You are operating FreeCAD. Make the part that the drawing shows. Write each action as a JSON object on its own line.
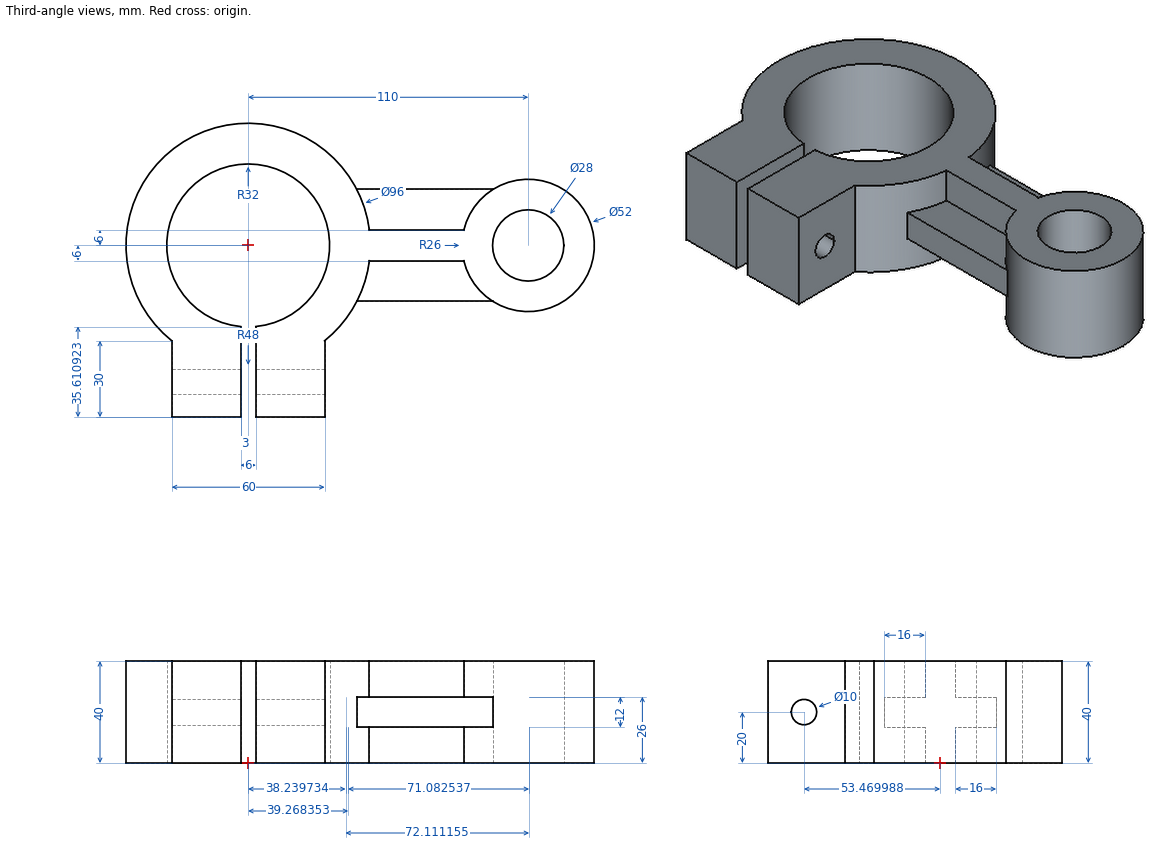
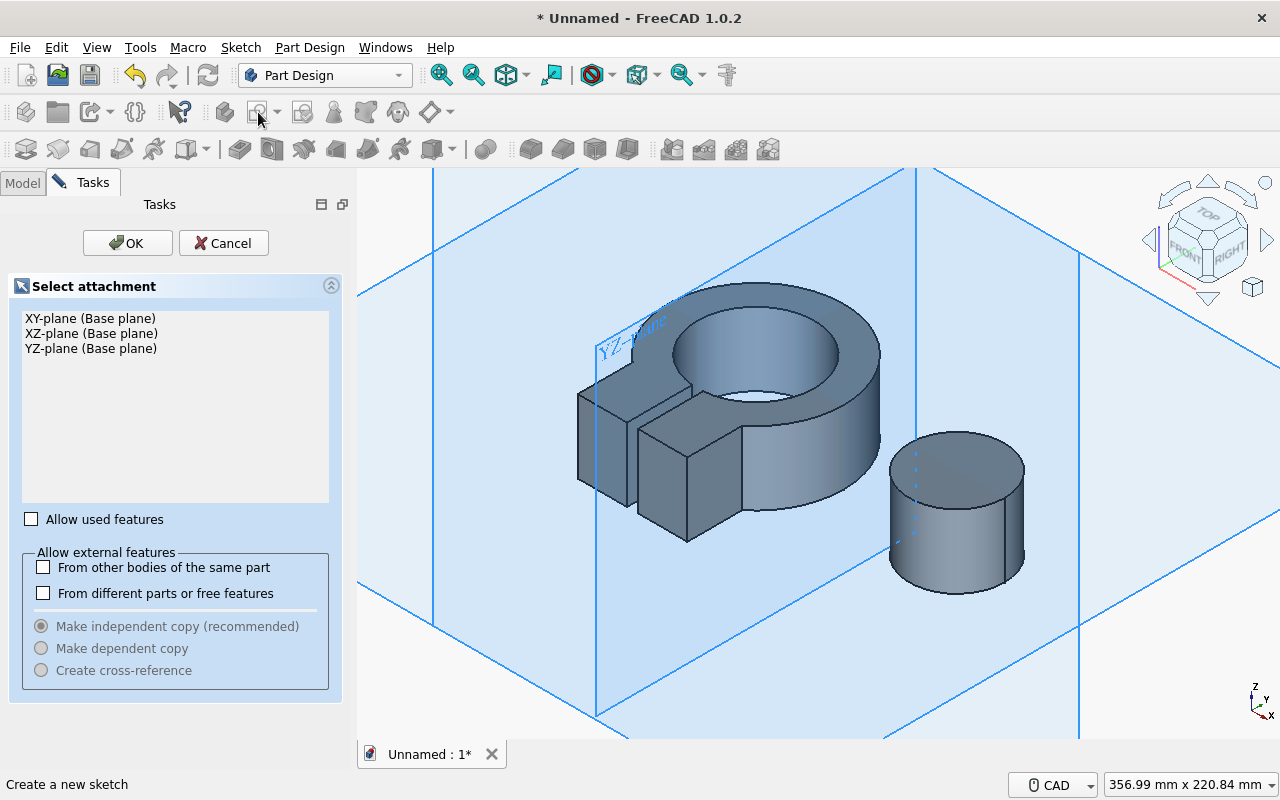
{"action": "left_click", "coordinate": [82, 318]}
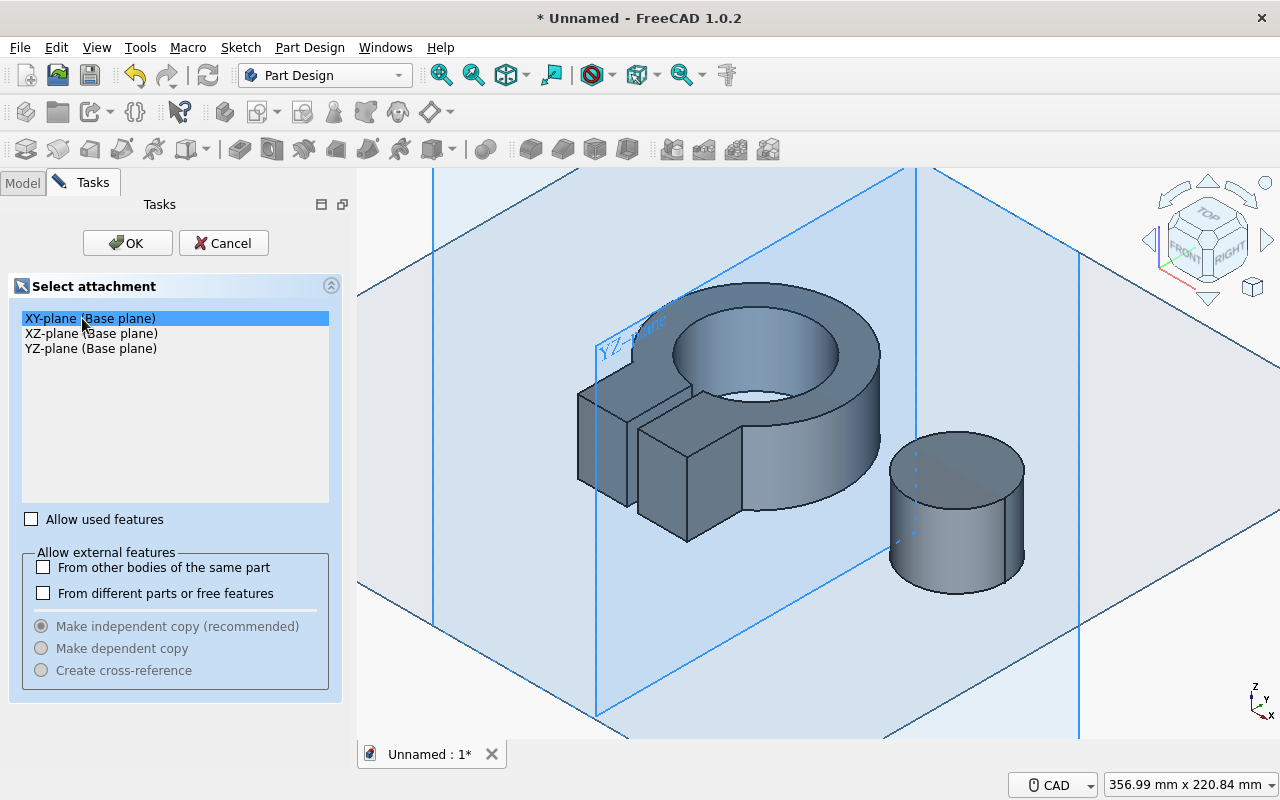
{"action": "left_click", "coordinate": [128, 243]}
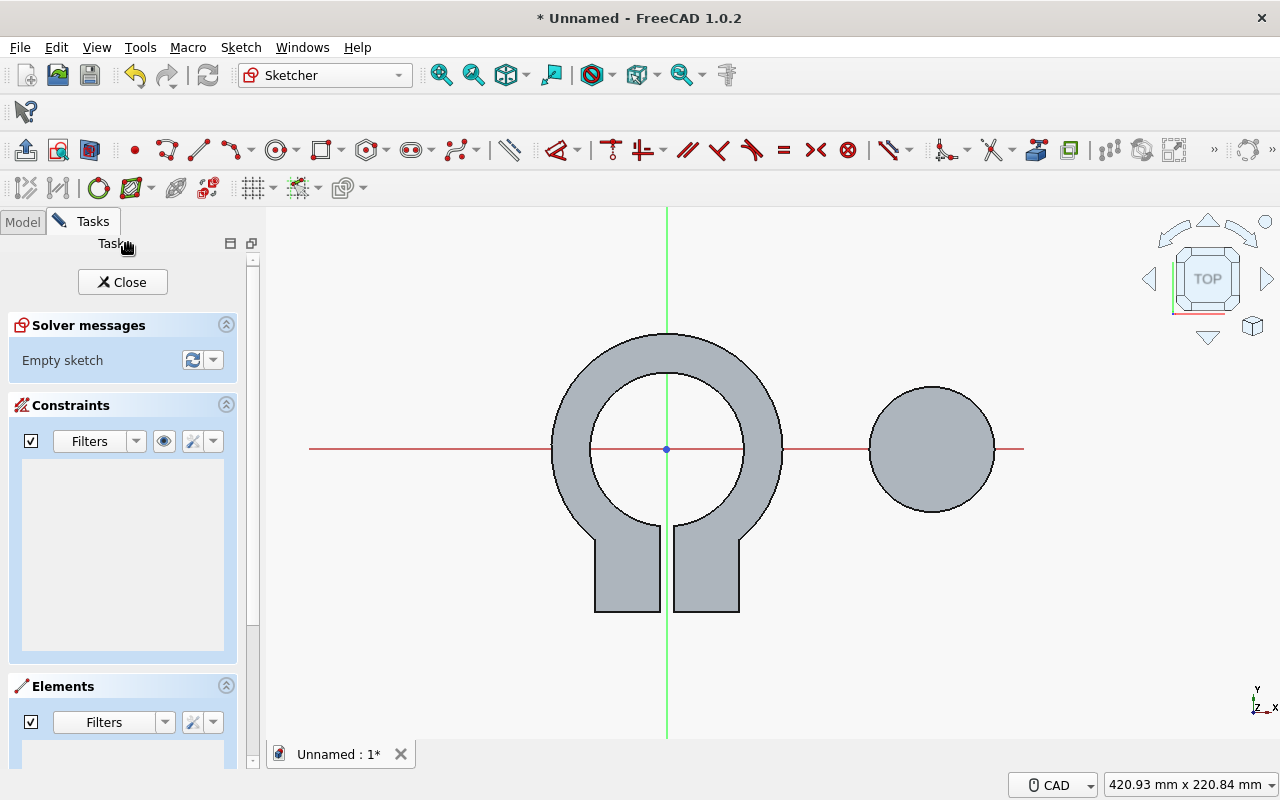
{"action": "left_click", "coordinate": [90, 150]}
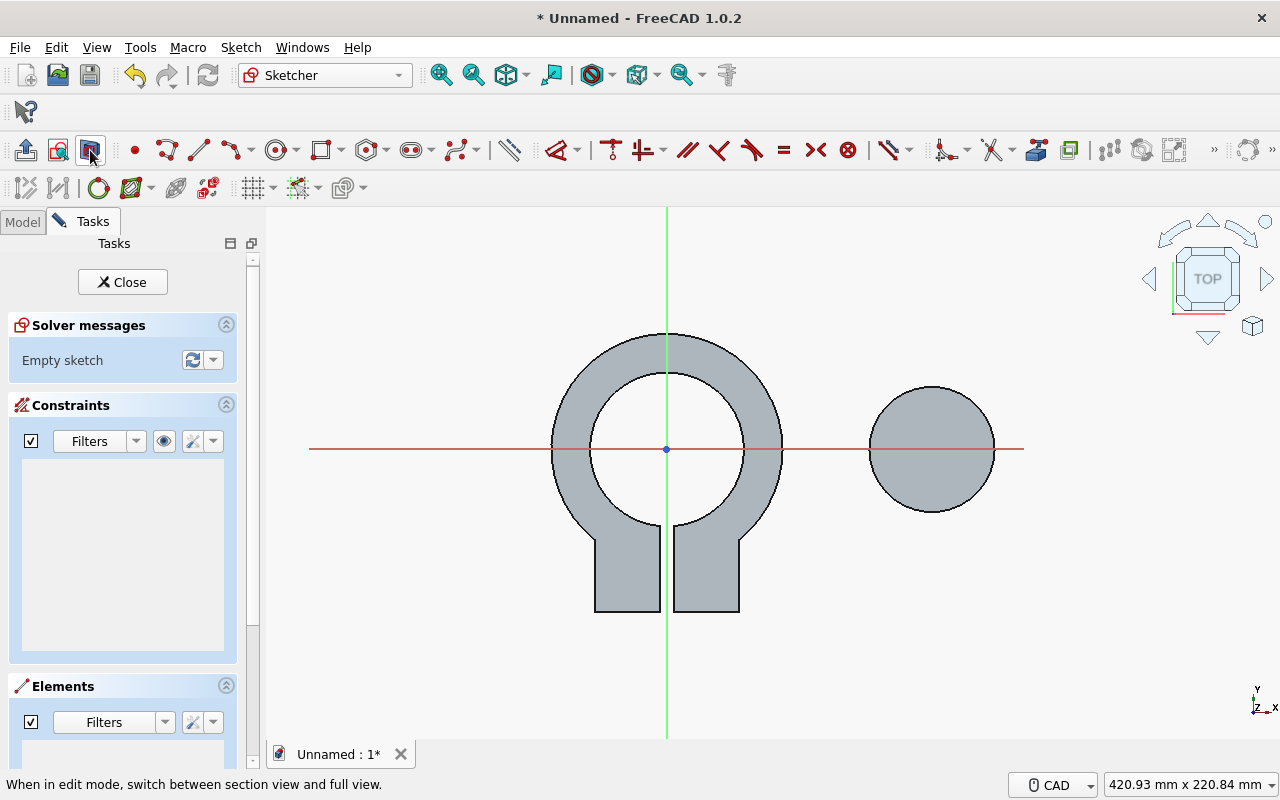
{"action": "scroll", "coordinate": [807, 436], "scroll_direction": "up", "scroll_amount": 5}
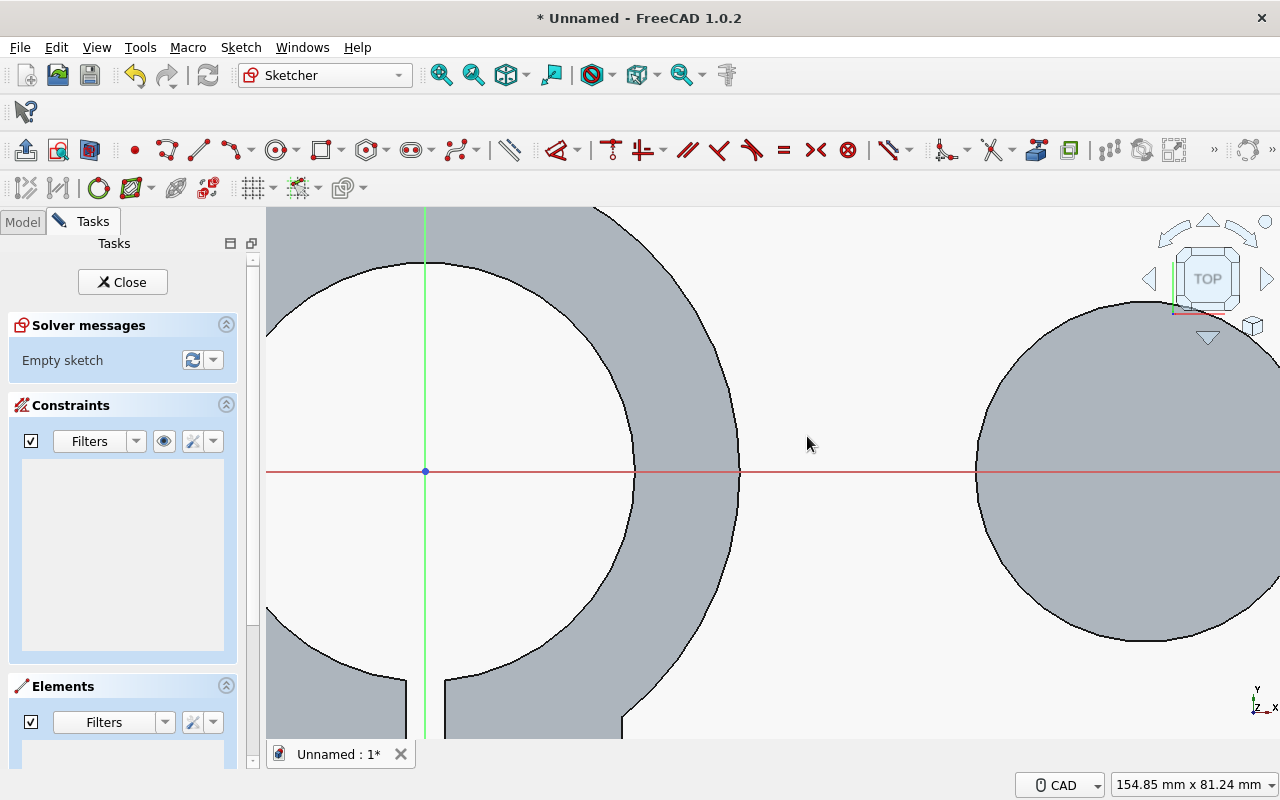
{"action": "left_click", "coordinate": [200, 150]}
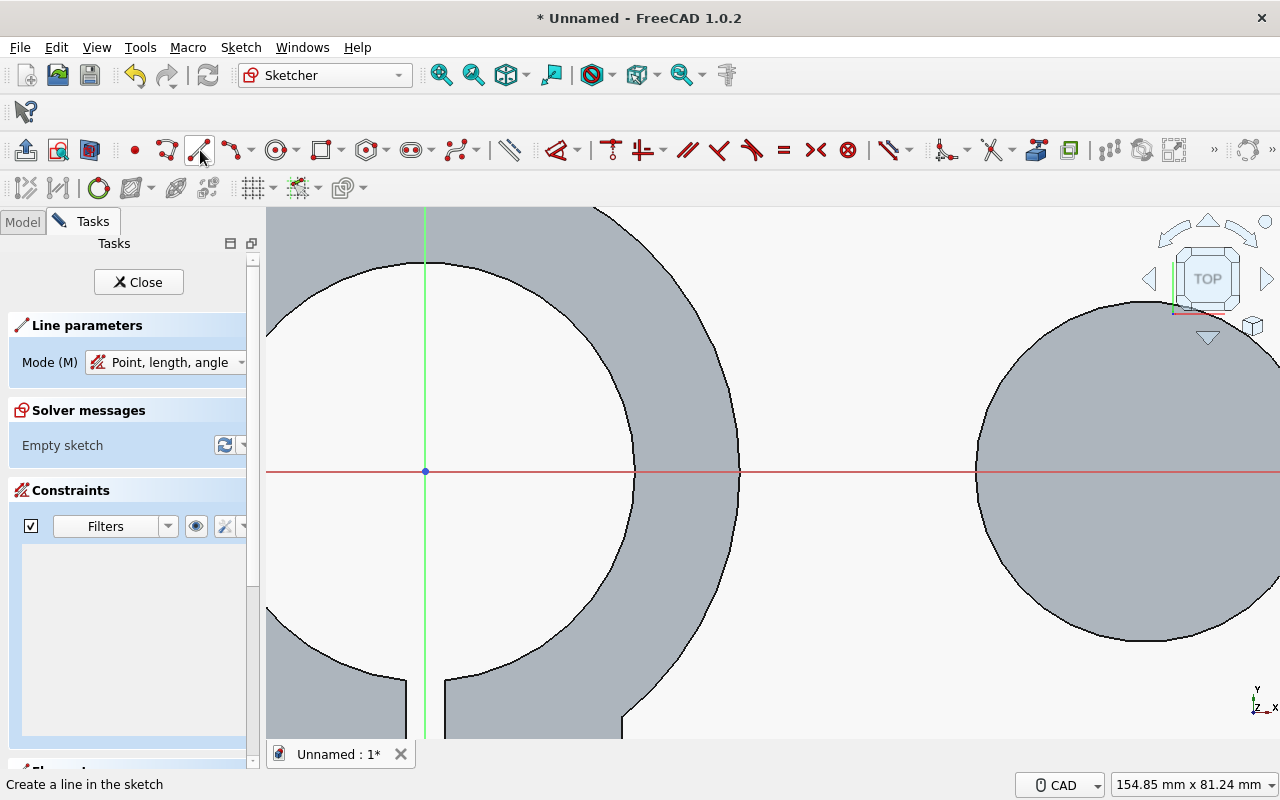
{"action": "left_click", "coordinate": [980, 433]}
{"action": "left_click", "coordinate": [737, 433]}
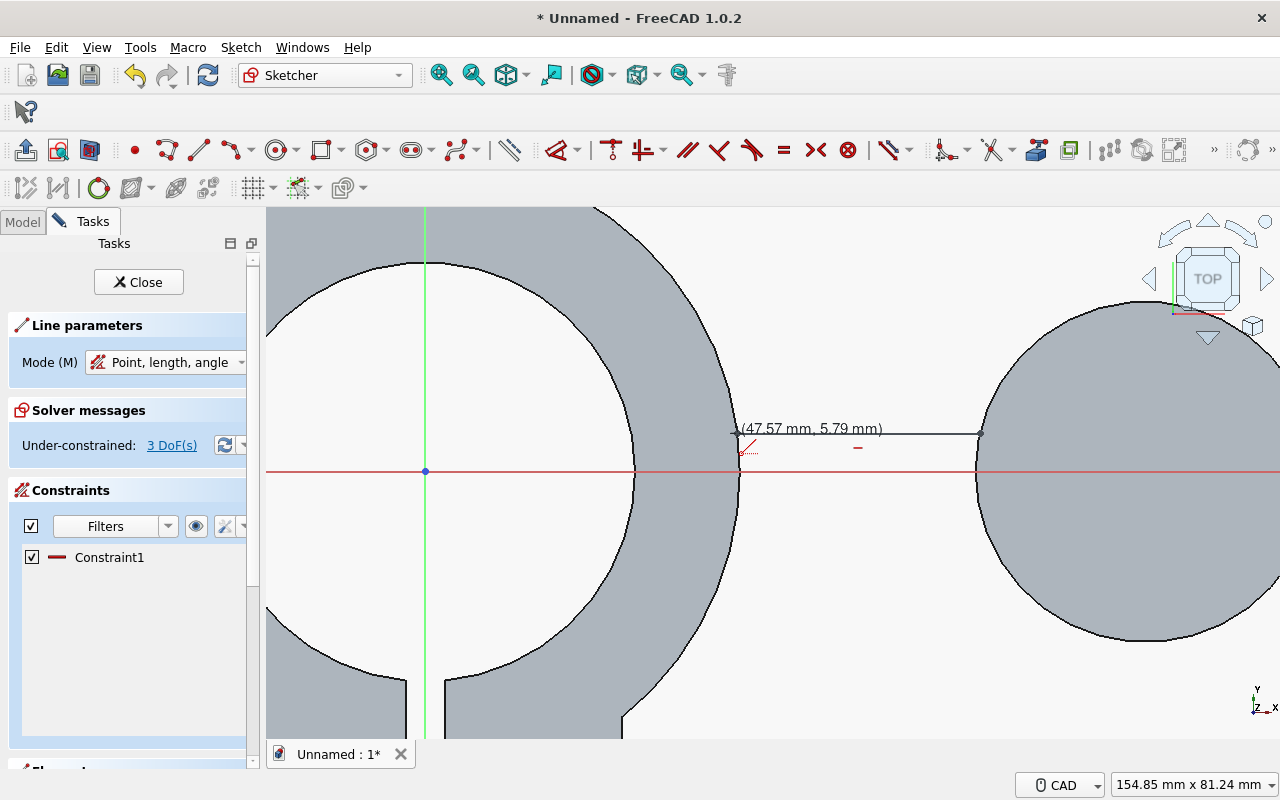
{"action": "left_click", "coordinate": [737, 511]}
{"action": "left_click", "coordinate": [980, 511]}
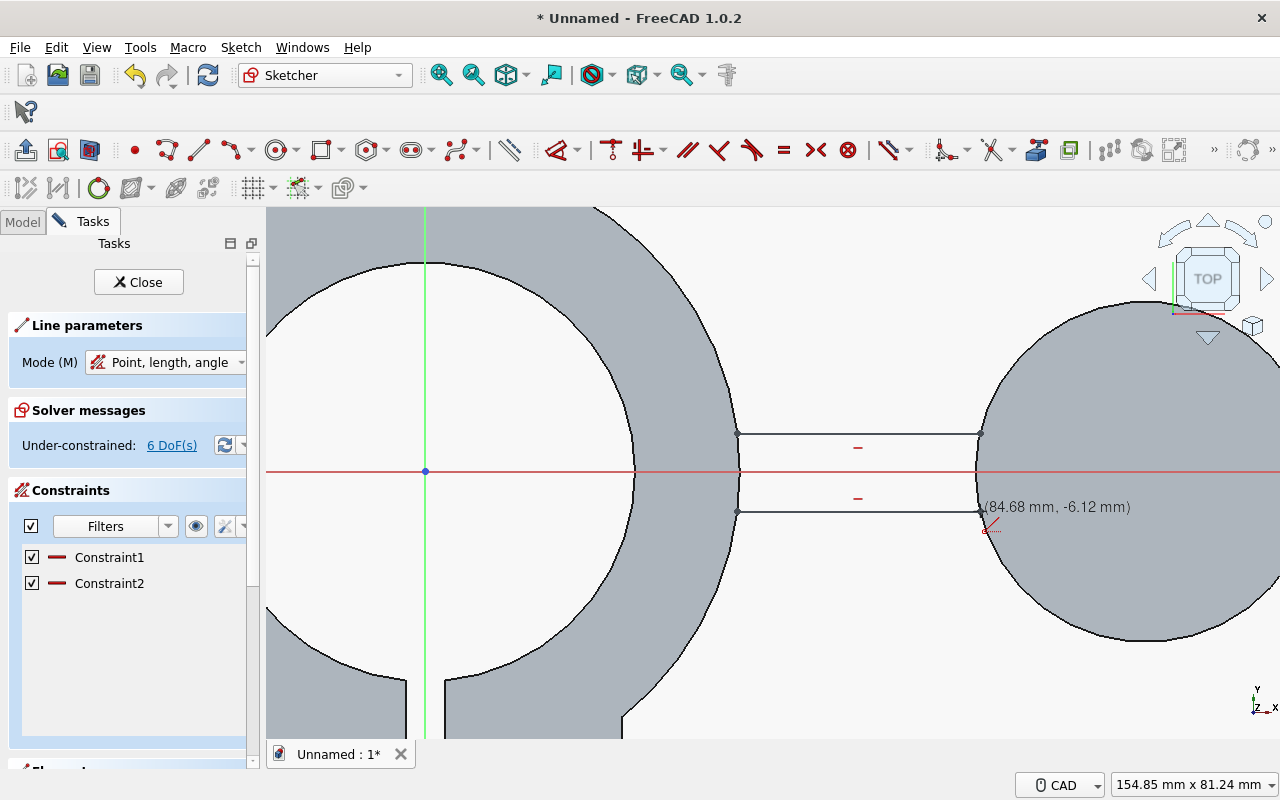
{"action": "left_click", "coordinate": [232, 150]}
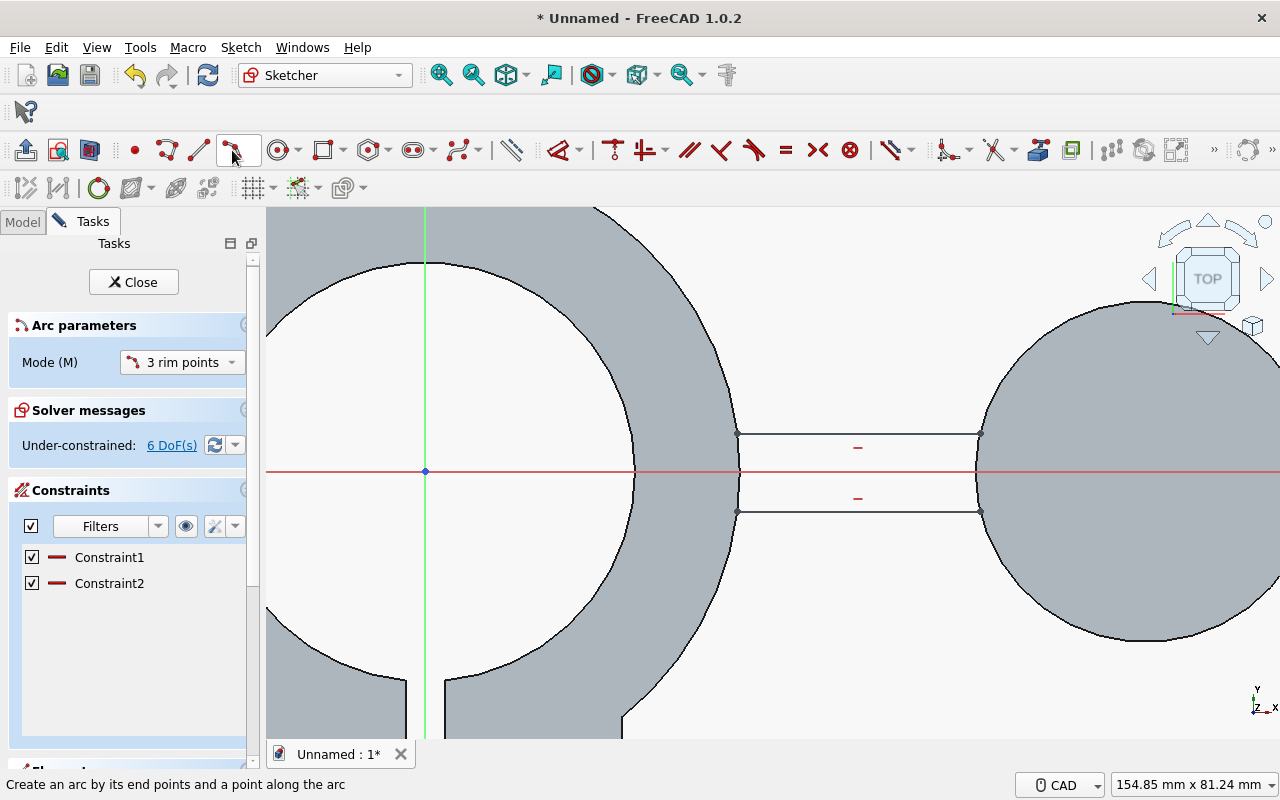
{"action": "left_click", "coordinate": [737, 434]}
{"action": "left_click", "coordinate": [737, 512]}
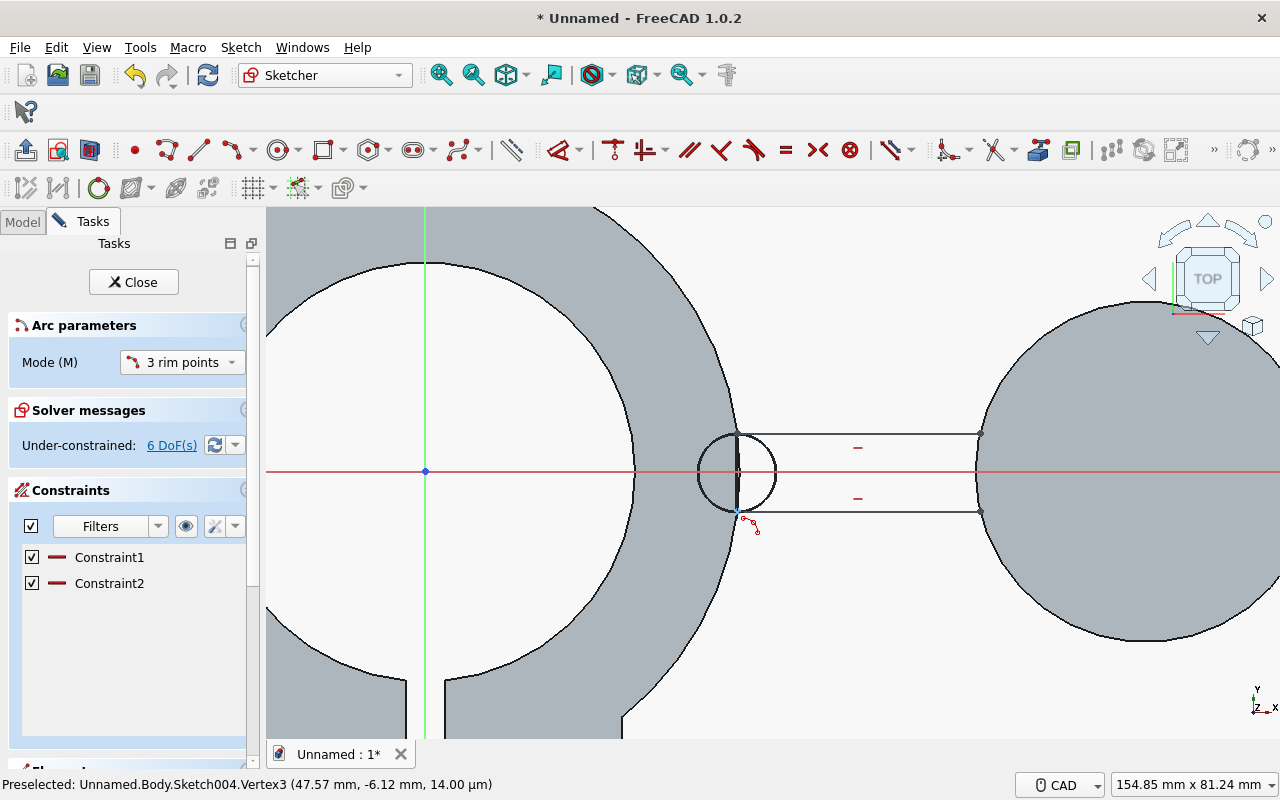
{"action": "scroll", "coordinate": [740, 480], "scroll_direction": "up", "scroll_amount": 10}